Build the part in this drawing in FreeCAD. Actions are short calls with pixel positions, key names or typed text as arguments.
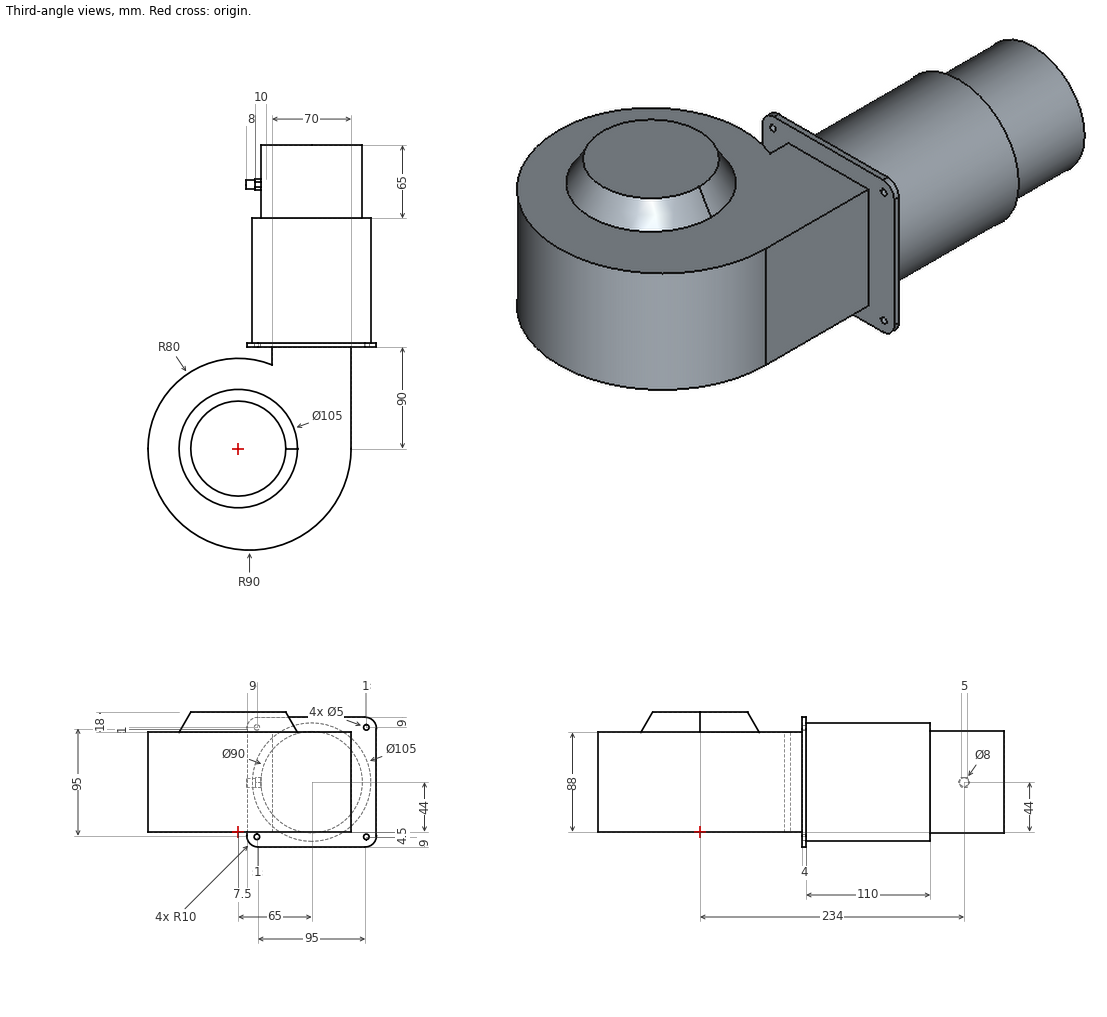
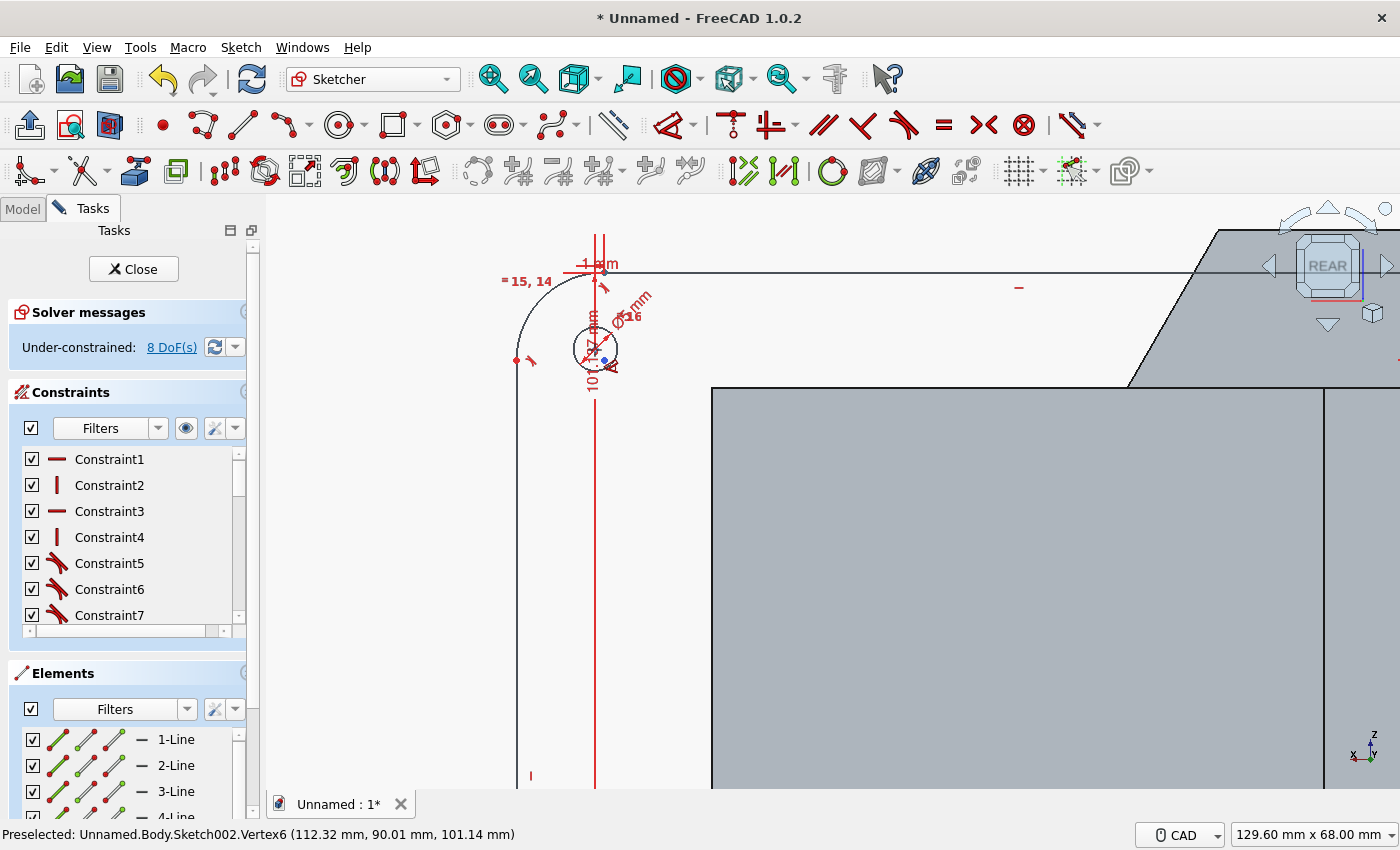
click(595, 349)
click(561, 311)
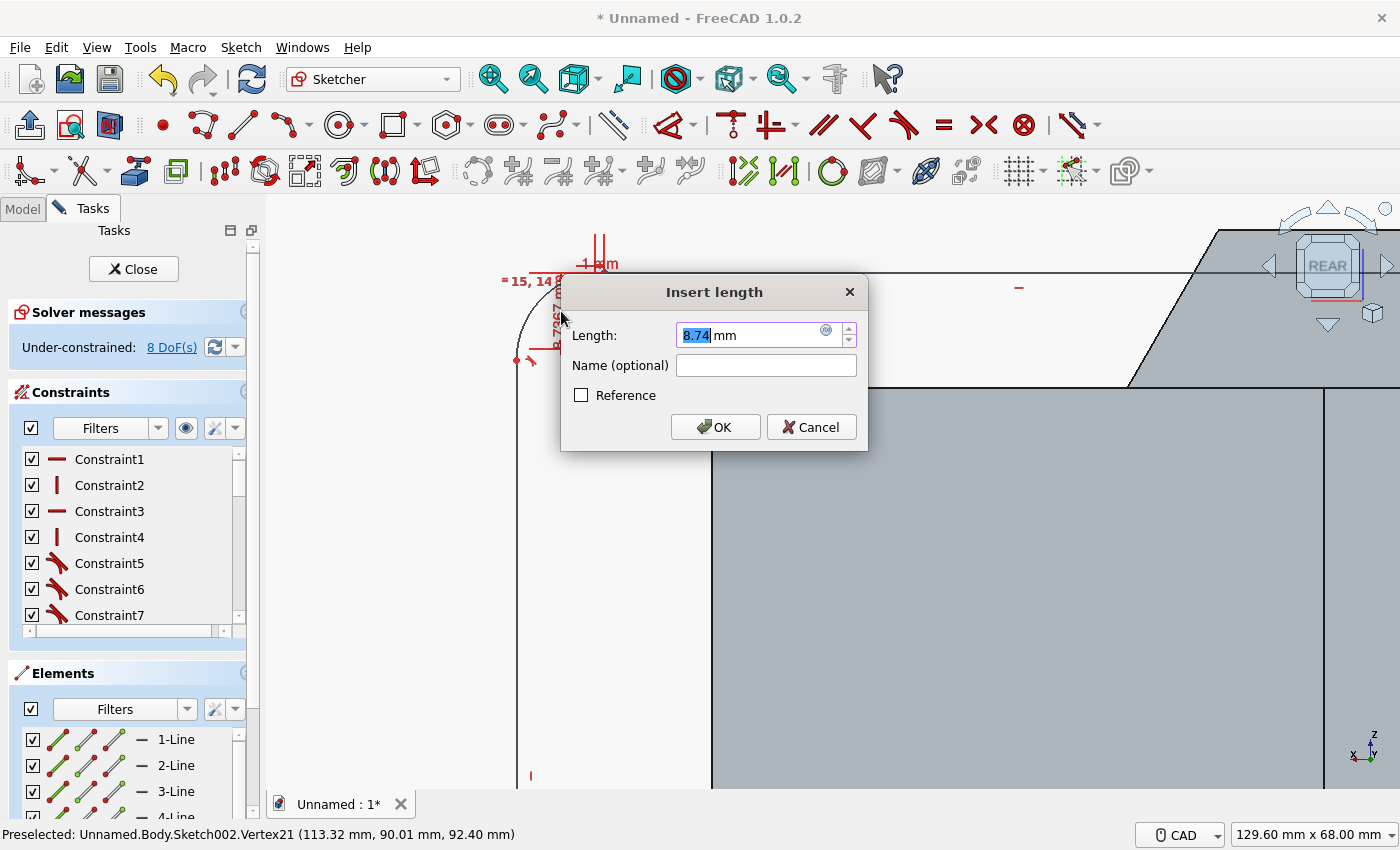
text(9)
key(Return)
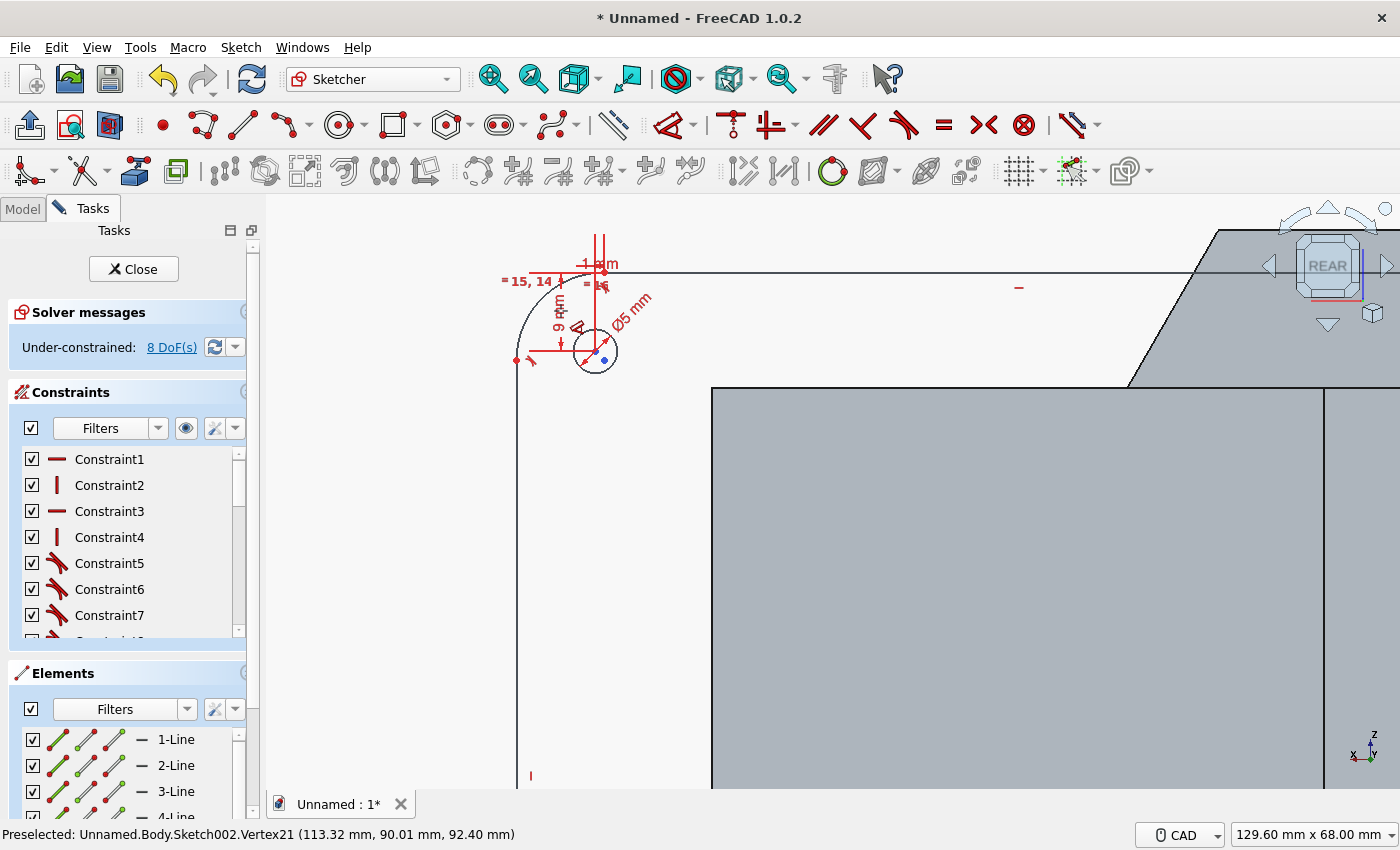
scroll(598, 328, down, 5)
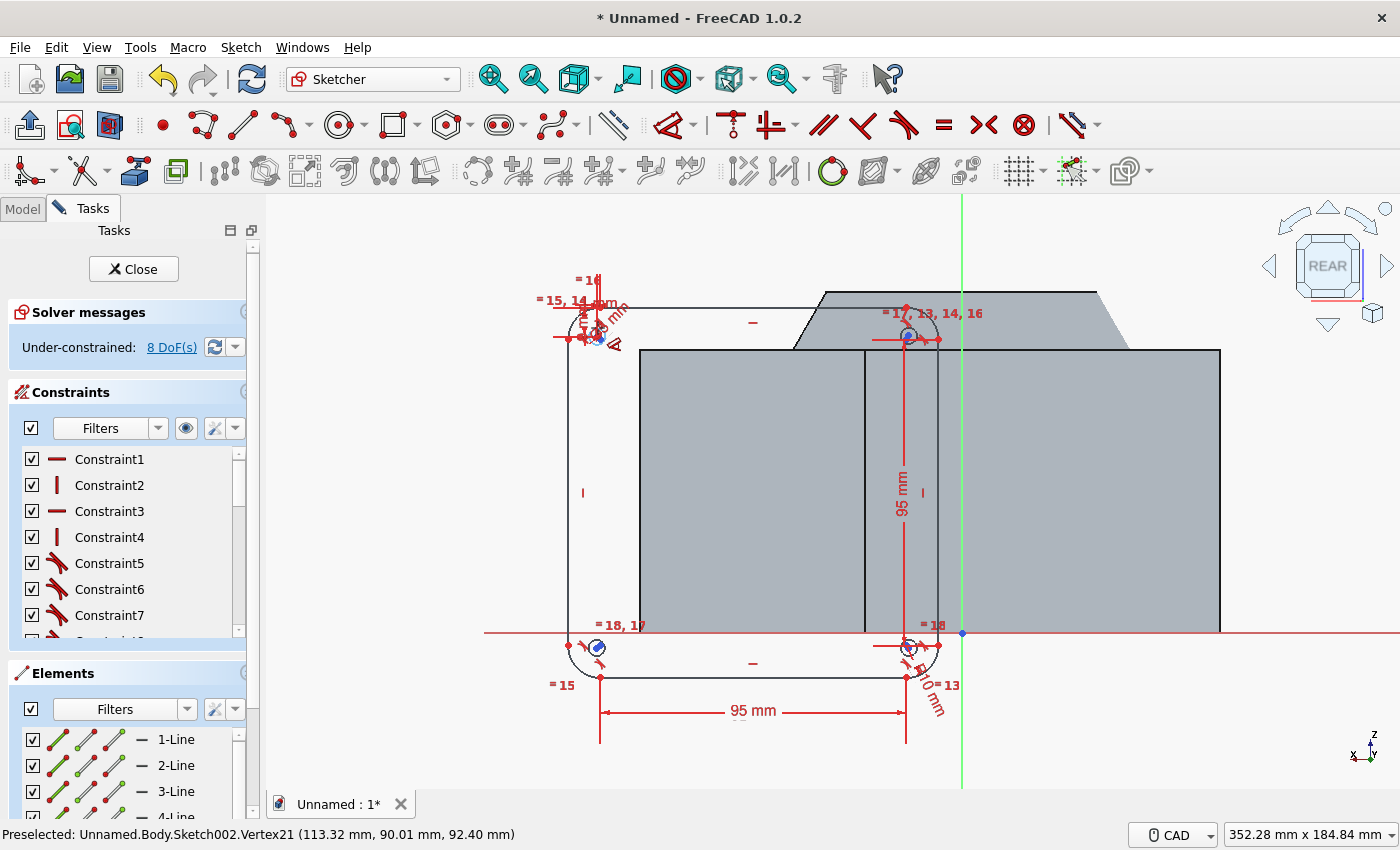
scroll(938, 340, up, 2)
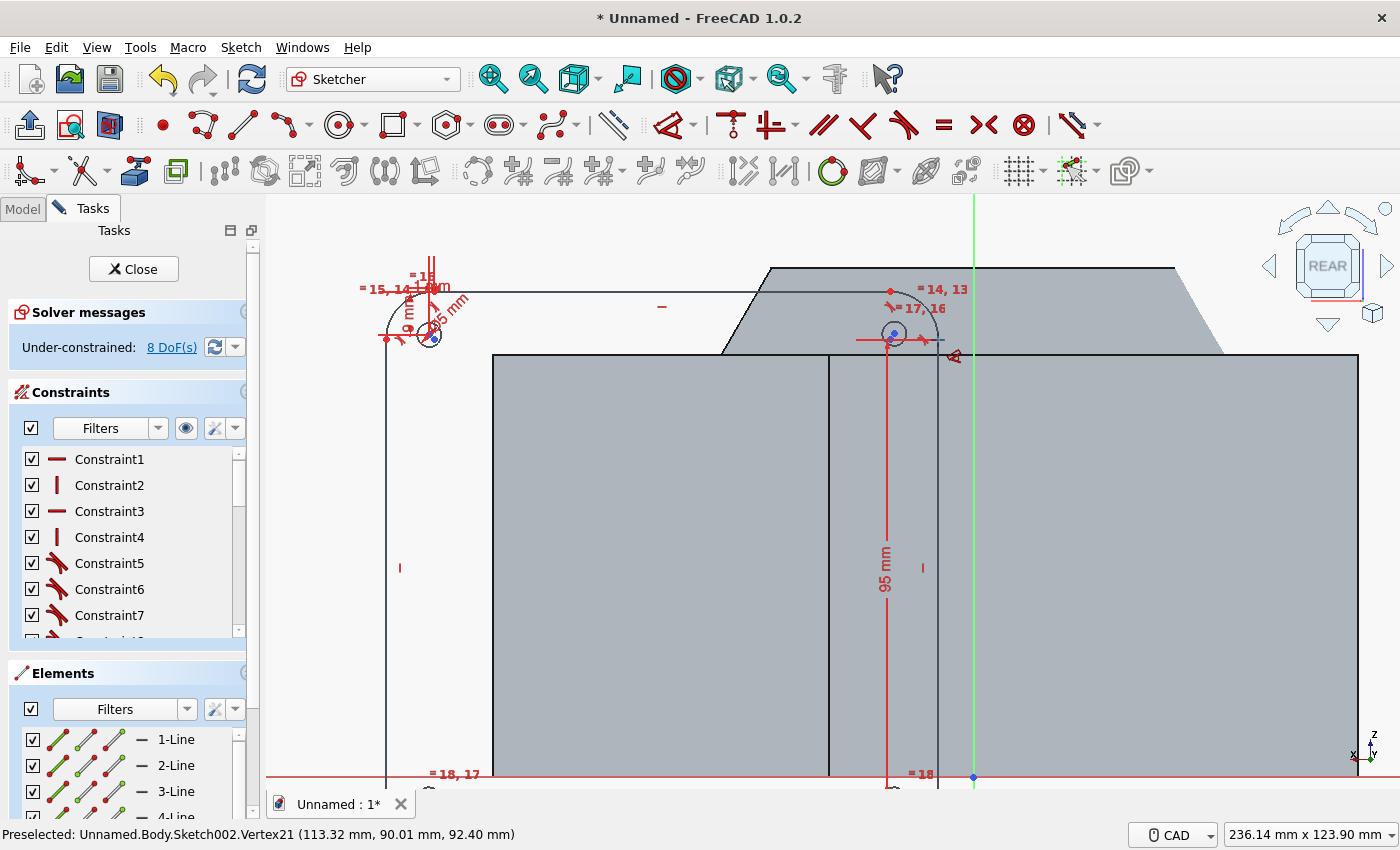
click(938, 340)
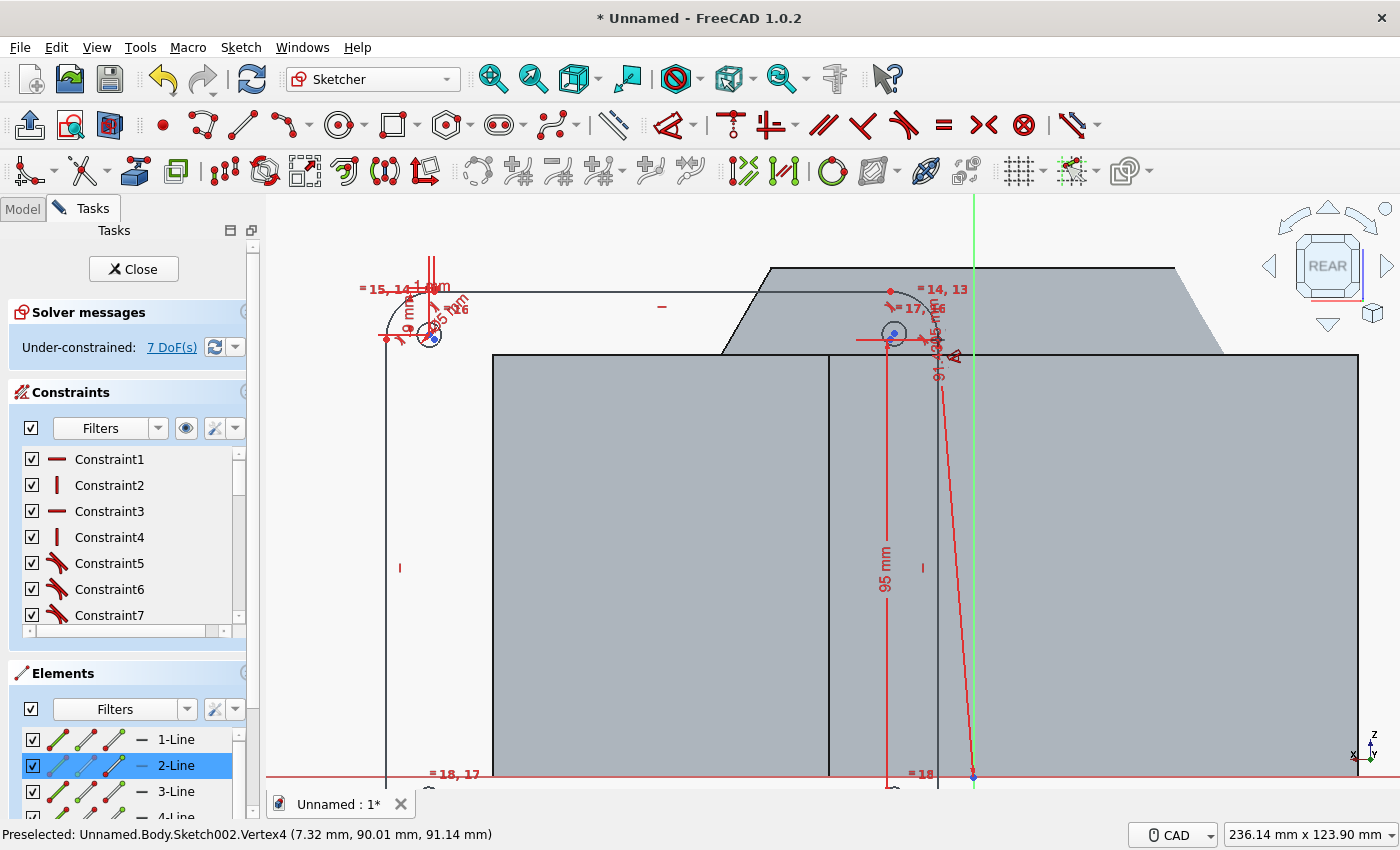
scroll(894, 334, up, 3)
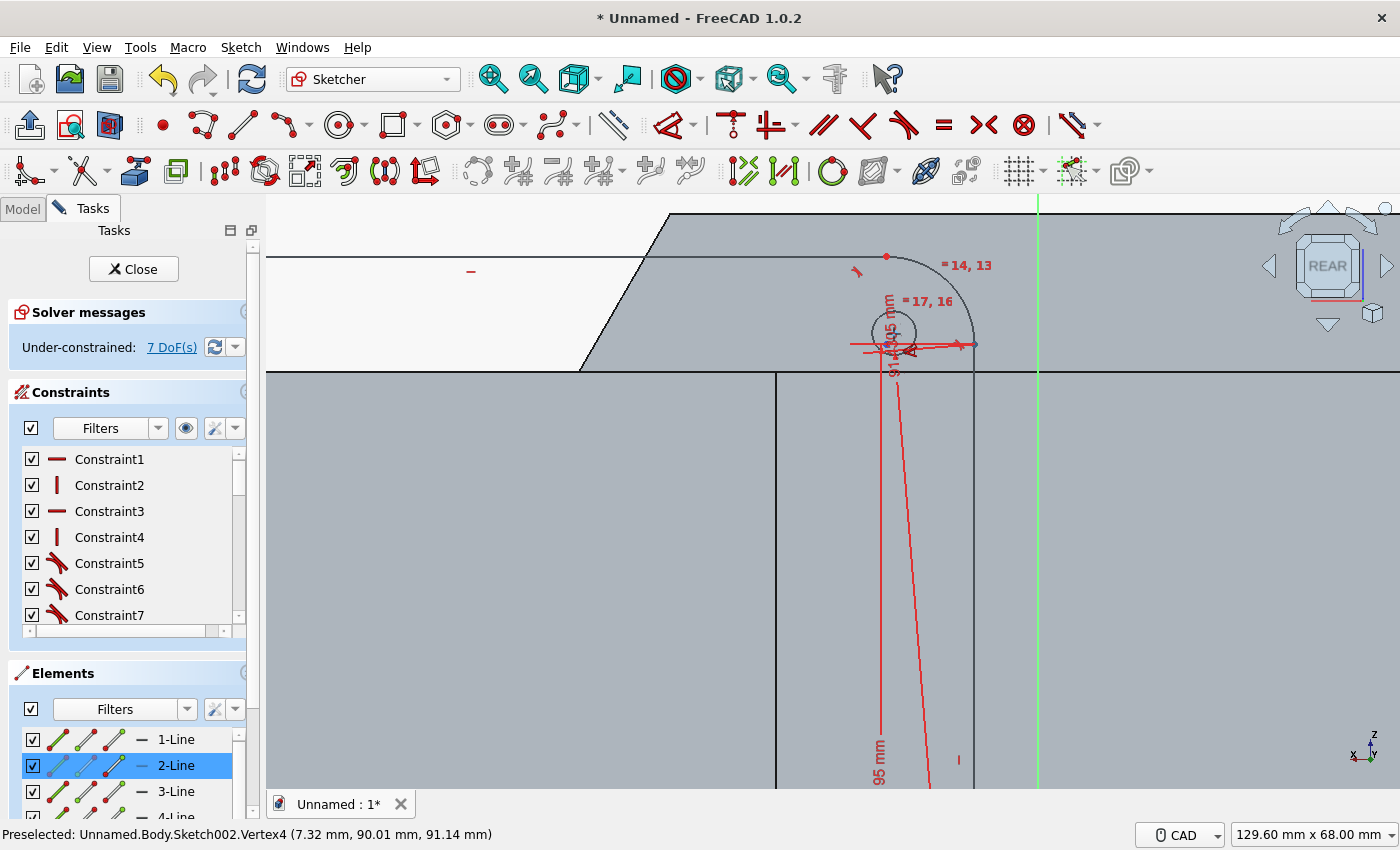
click(894, 333)
click(934, 299)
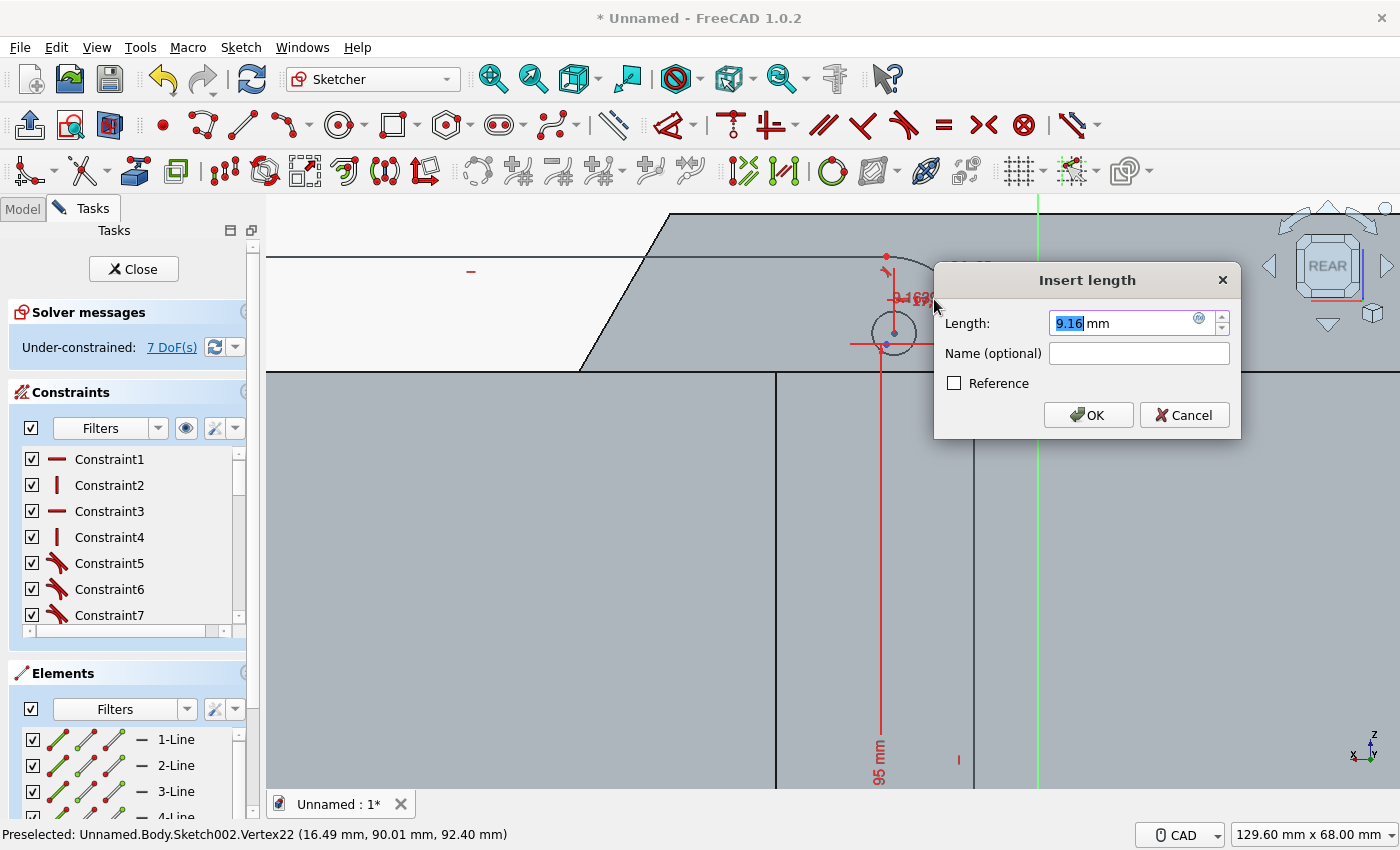
text(9)
key(Return)